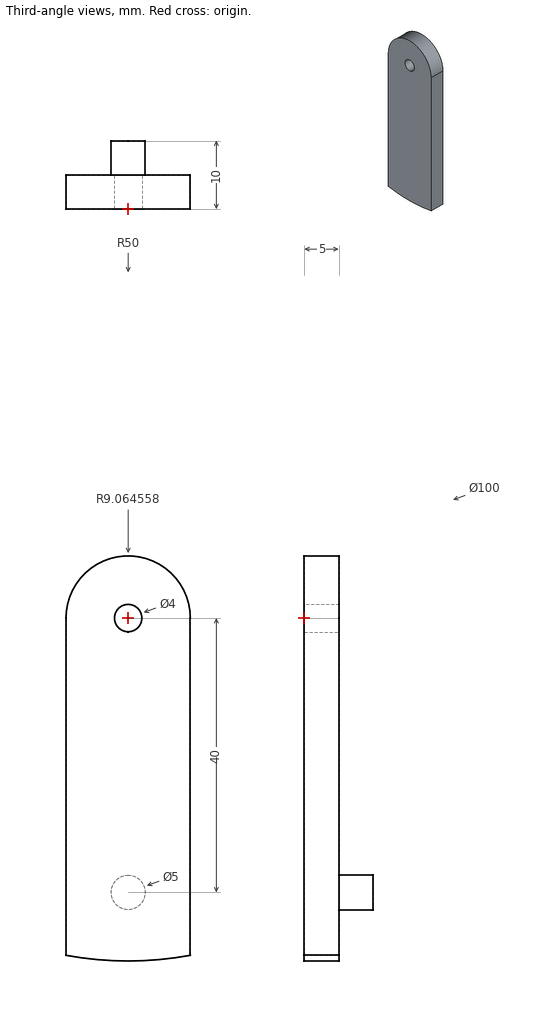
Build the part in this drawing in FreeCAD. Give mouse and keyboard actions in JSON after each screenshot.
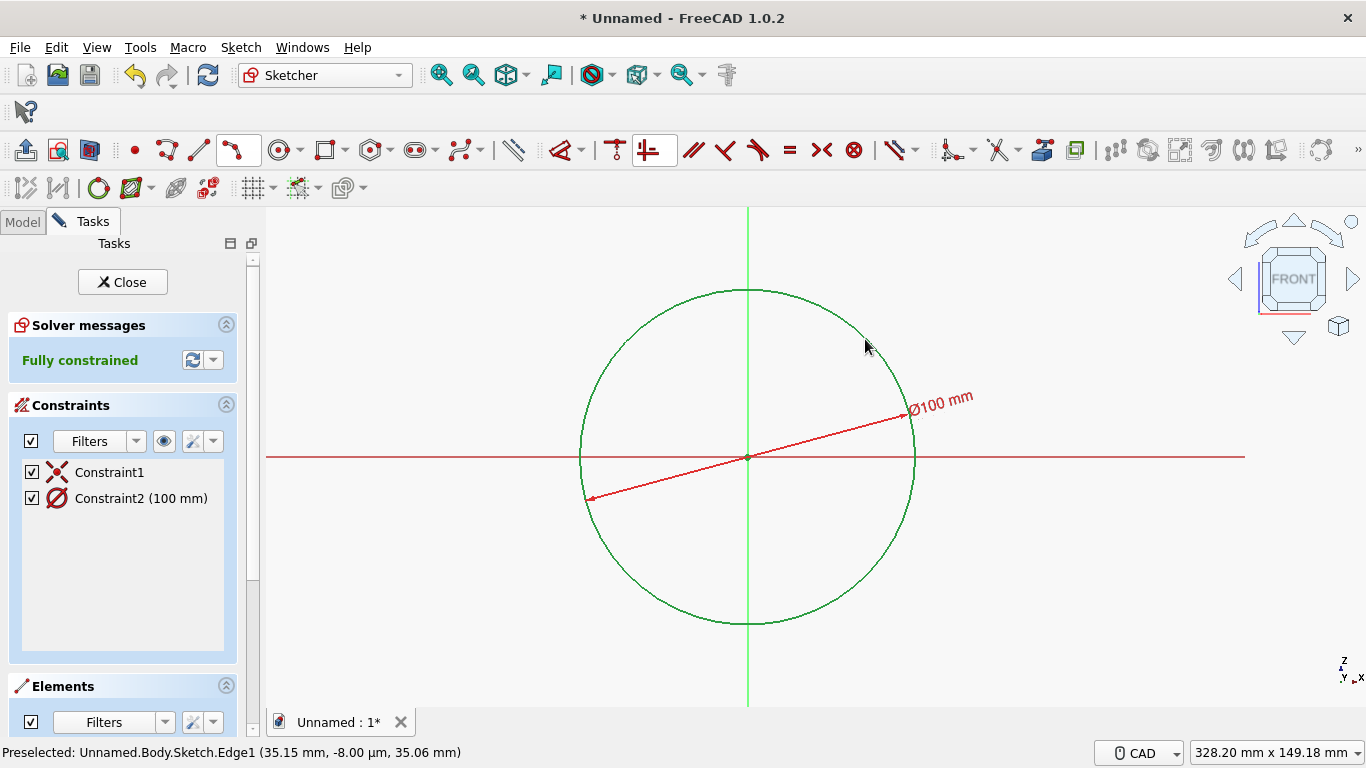
{"action": "left_click", "coordinate": [123, 282]}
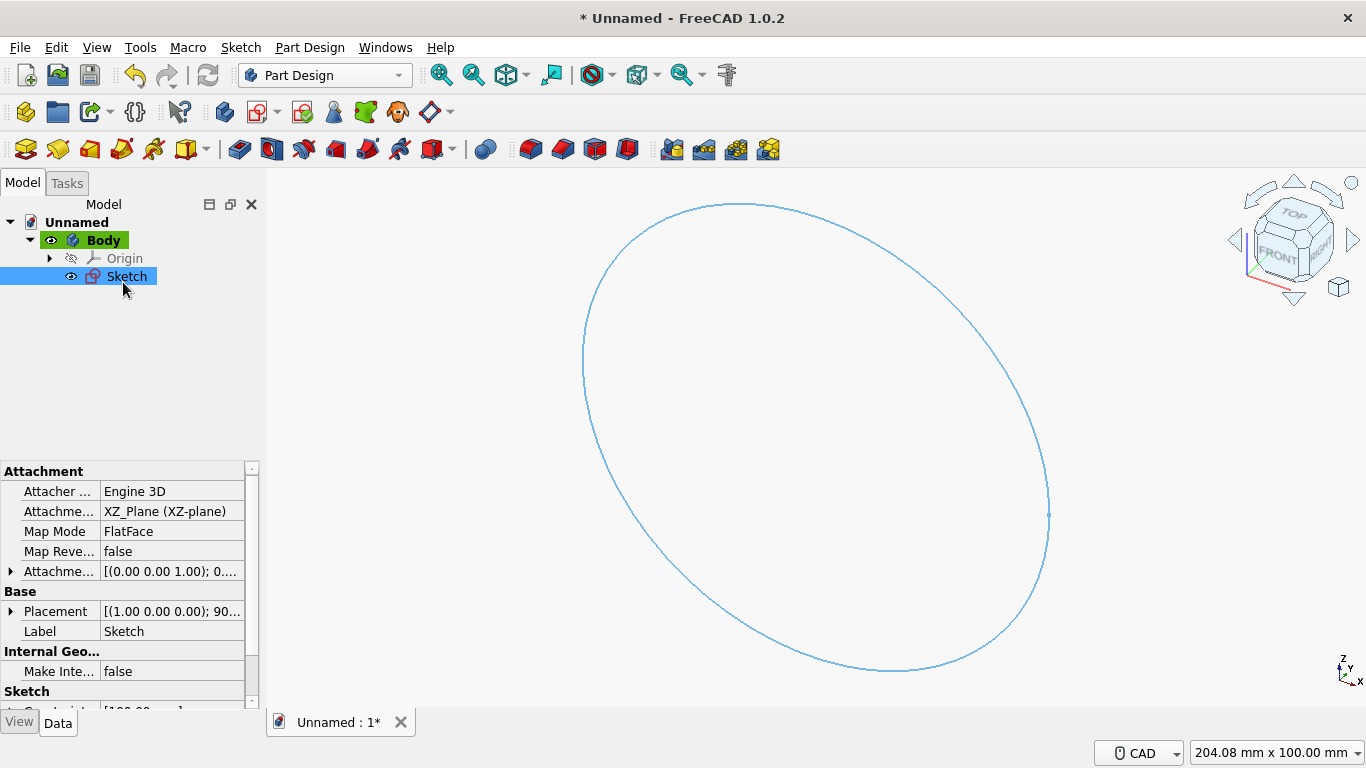
{"action": "left_click", "coordinate": [26, 150]}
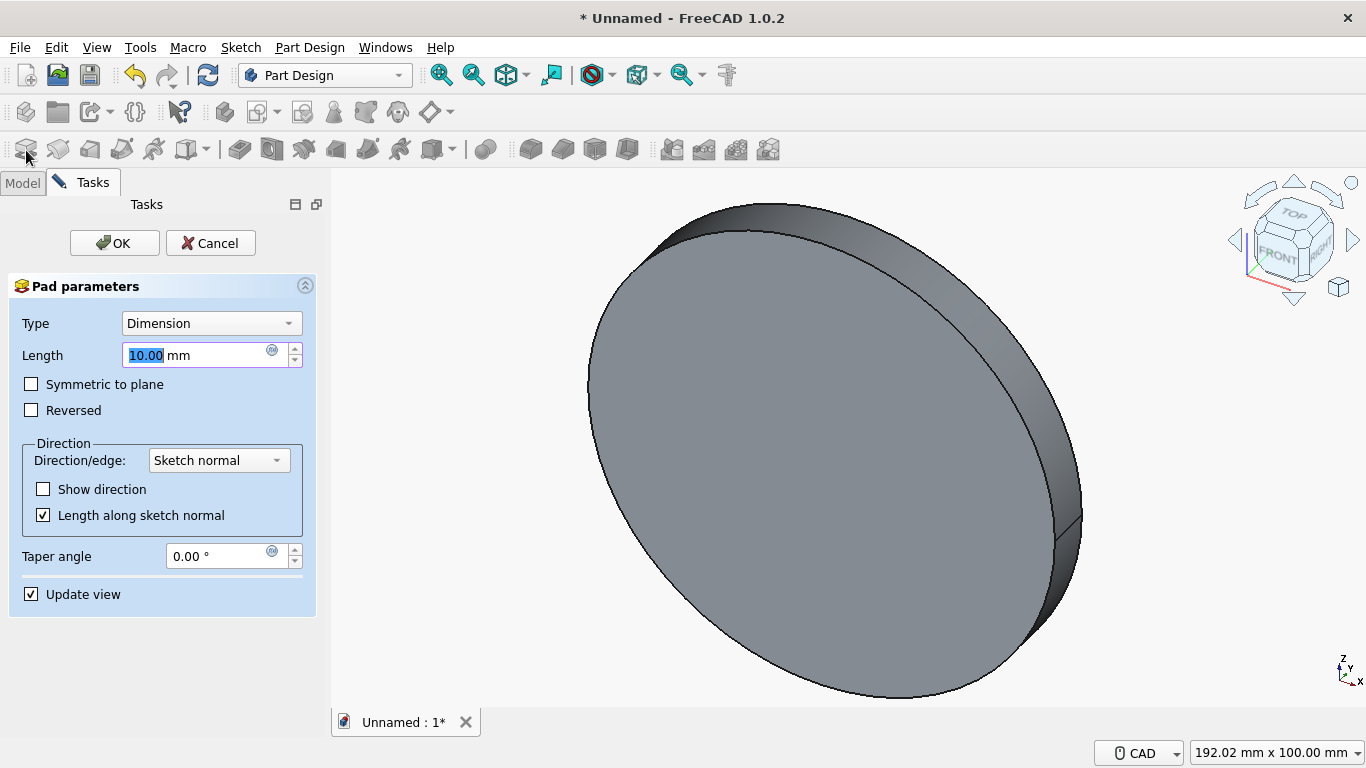
{"action": "type", "text": "5"}
{"action": "key", "text": "Tab"}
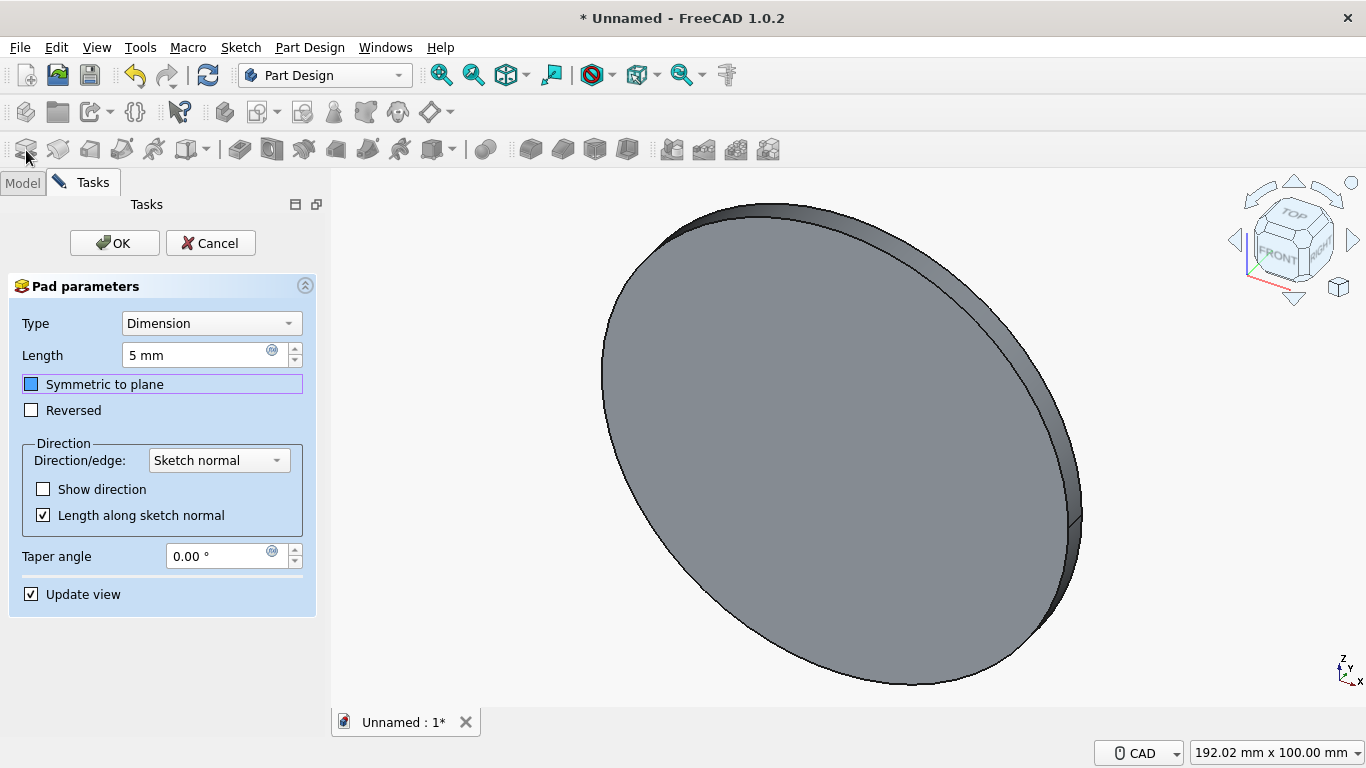
{"action": "left_click", "coordinate": [30, 410]}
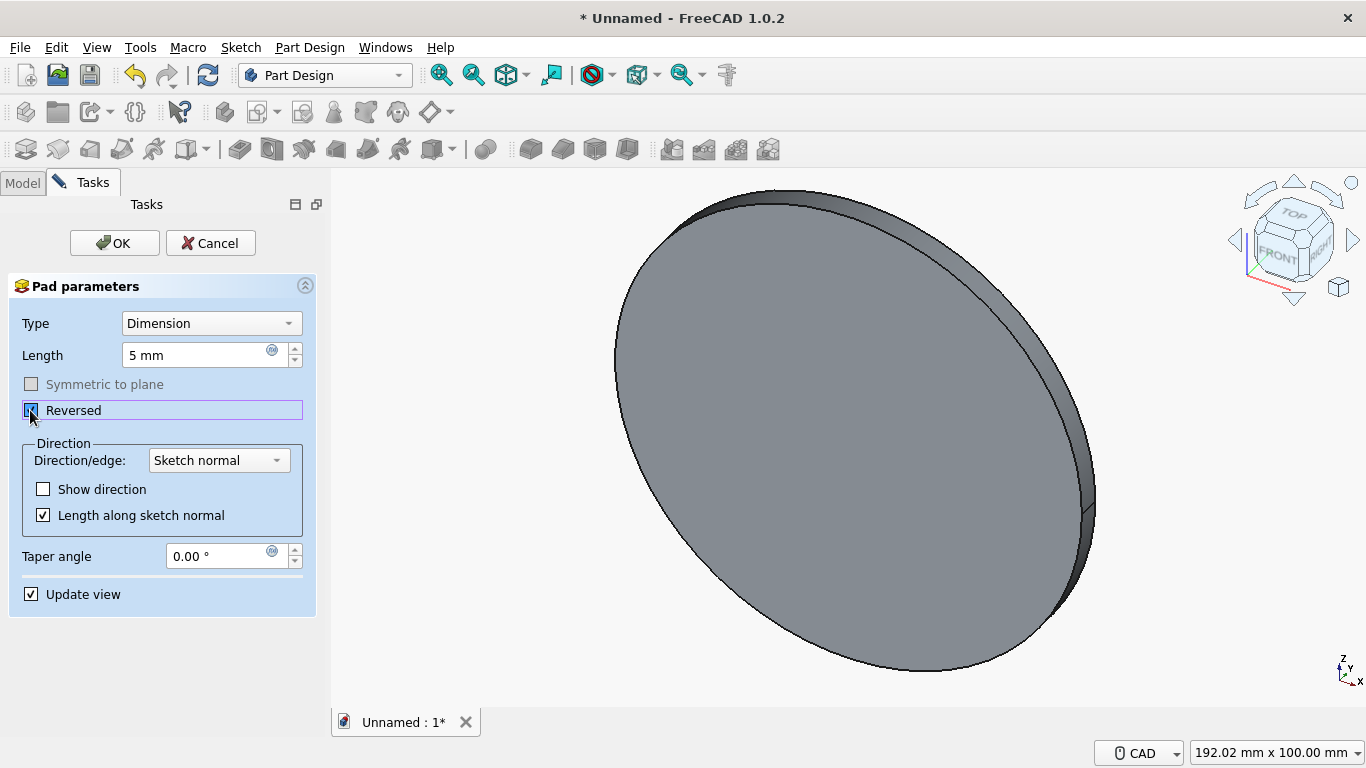
{"action": "left_click", "coordinate": [115, 243]}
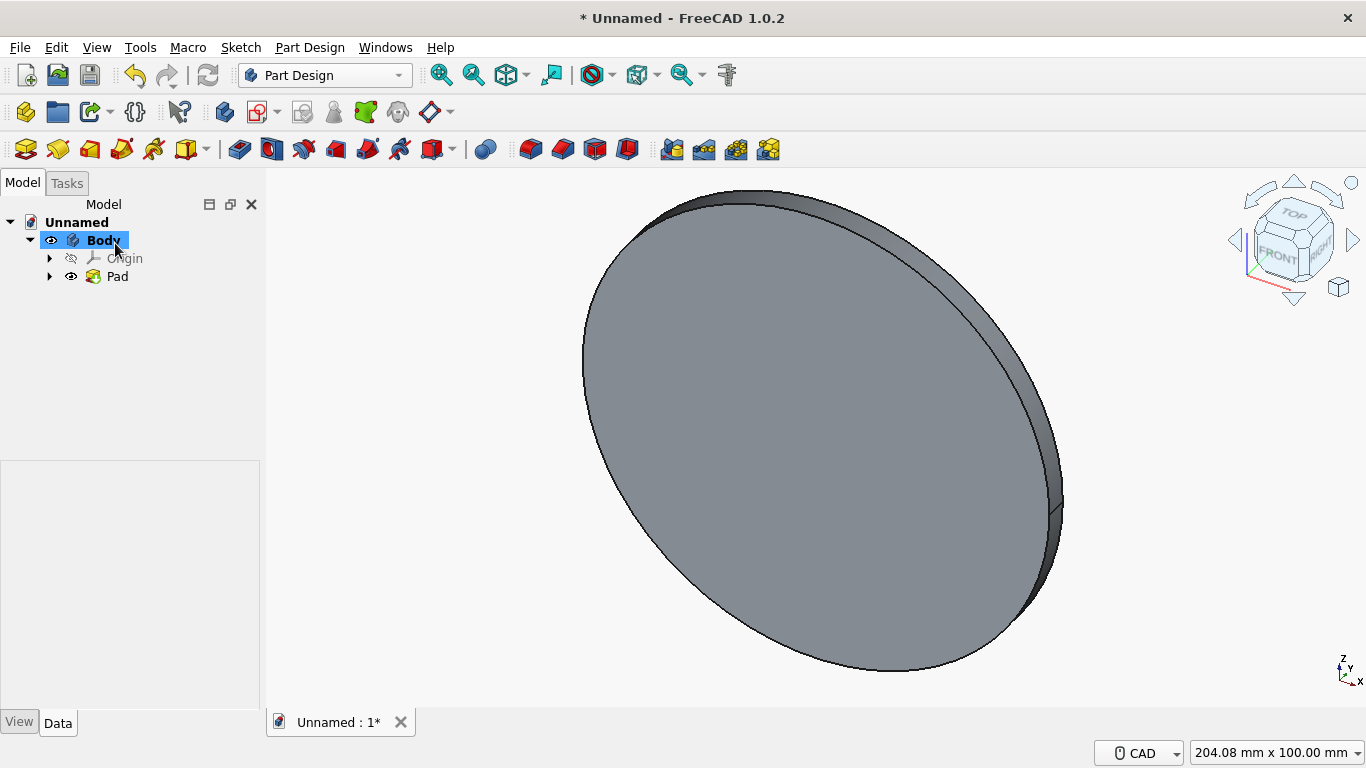
{"action": "left_click", "coordinate": [442, 76]}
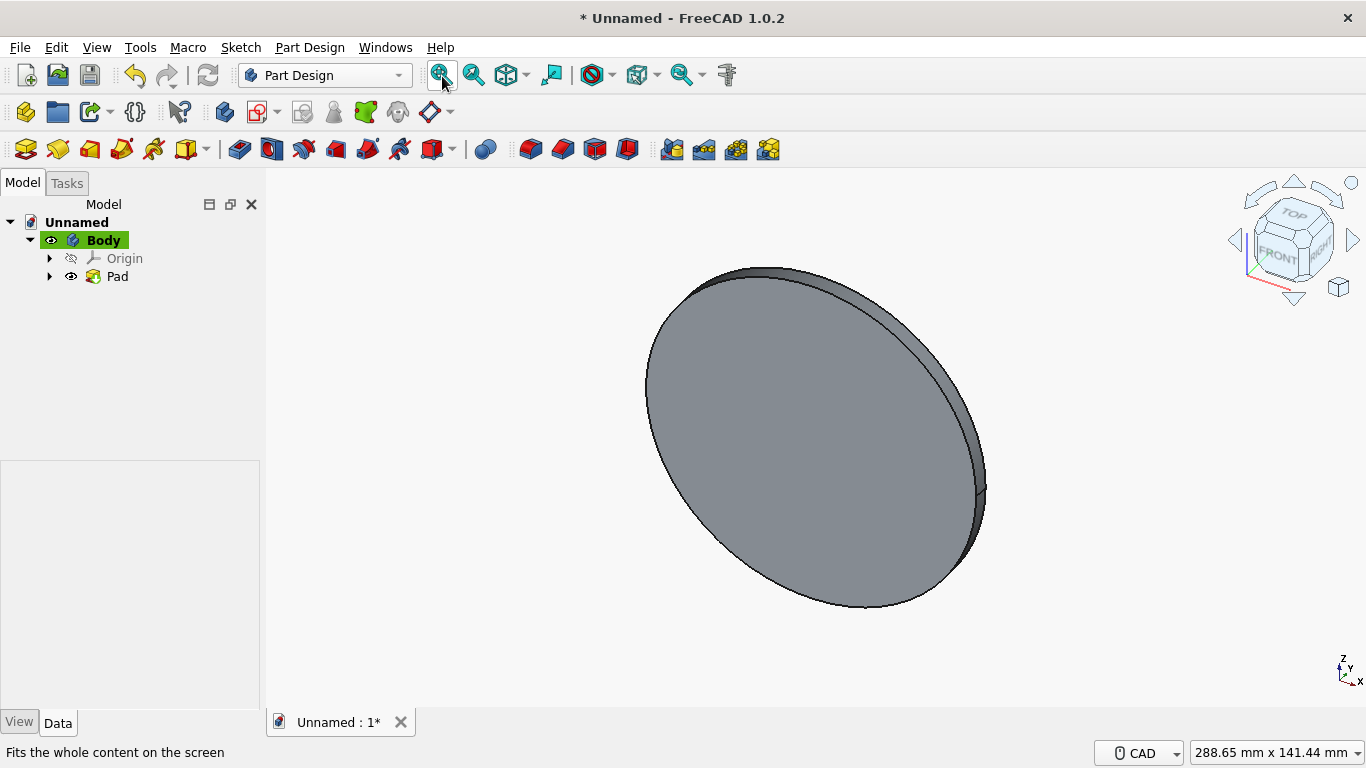
{"action": "left_click", "coordinate": [258, 112]}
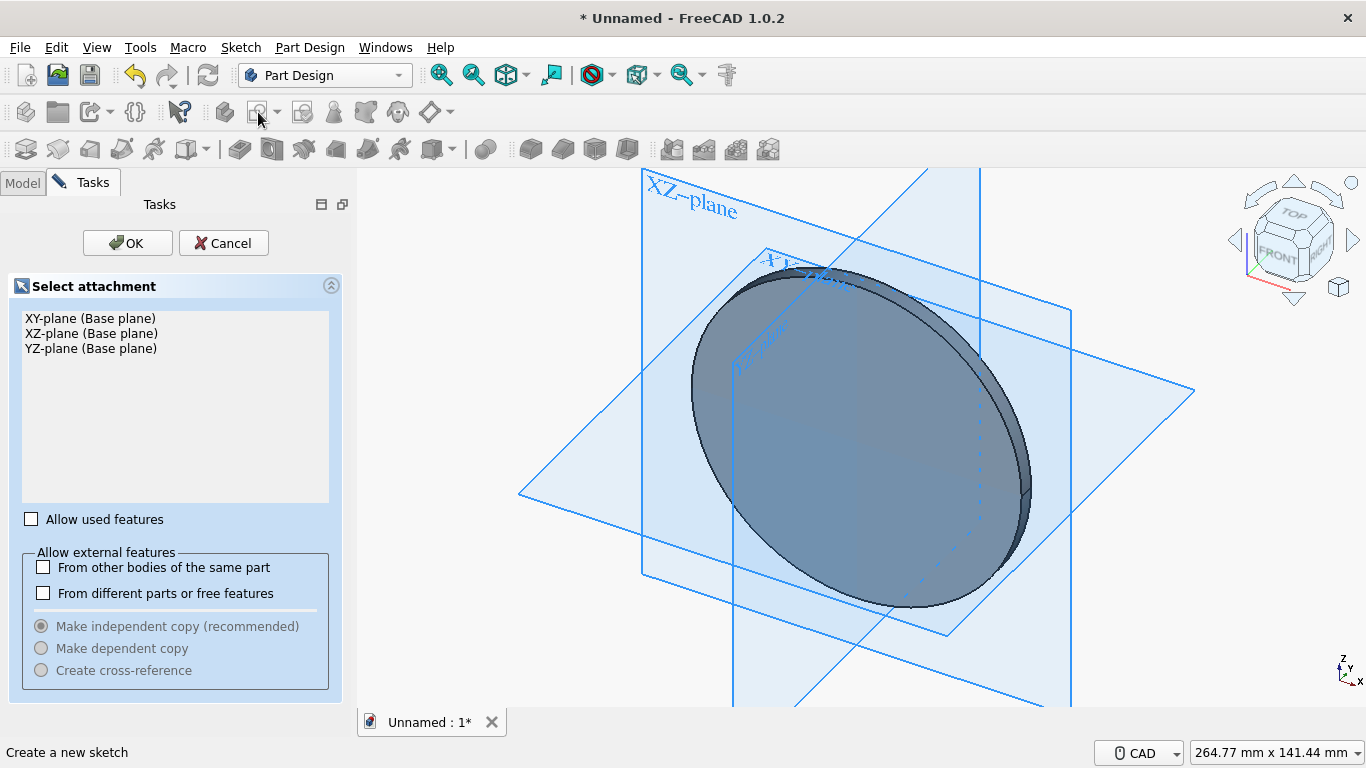
{"action": "left_click", "coordinate": [82, 334]}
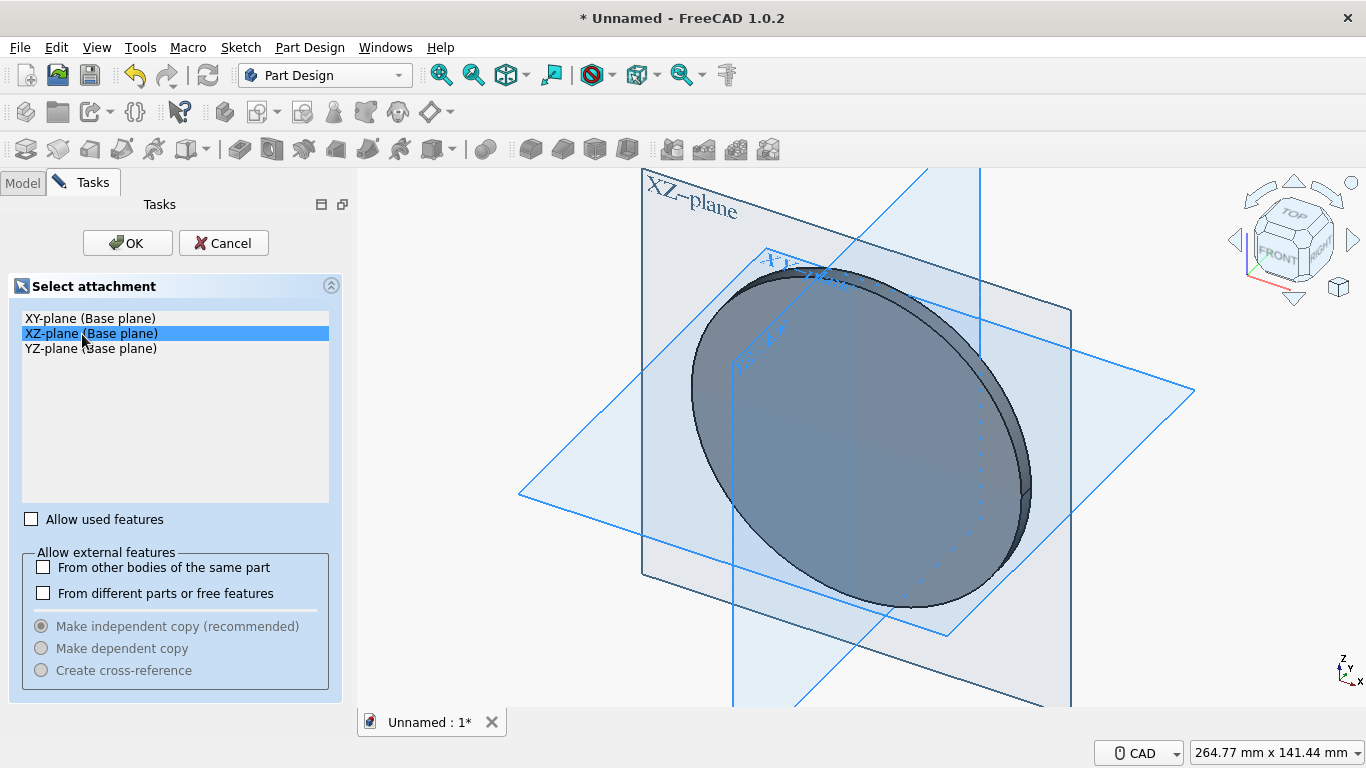
{"action": "left_click", "coordinate": [128, 243]}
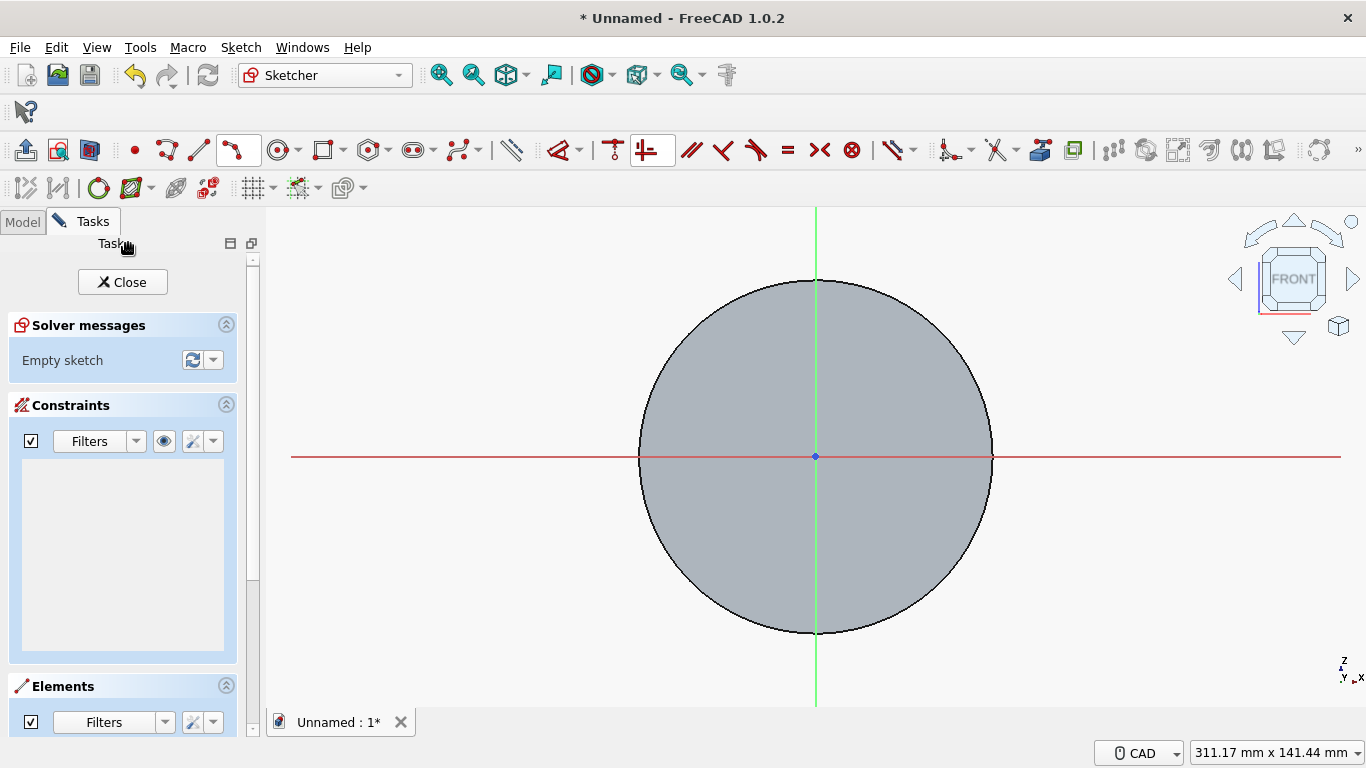
{"action": "scroll", "coordinate": [820, 608], "scroll_direction": "up", "scroll_amount": 14}